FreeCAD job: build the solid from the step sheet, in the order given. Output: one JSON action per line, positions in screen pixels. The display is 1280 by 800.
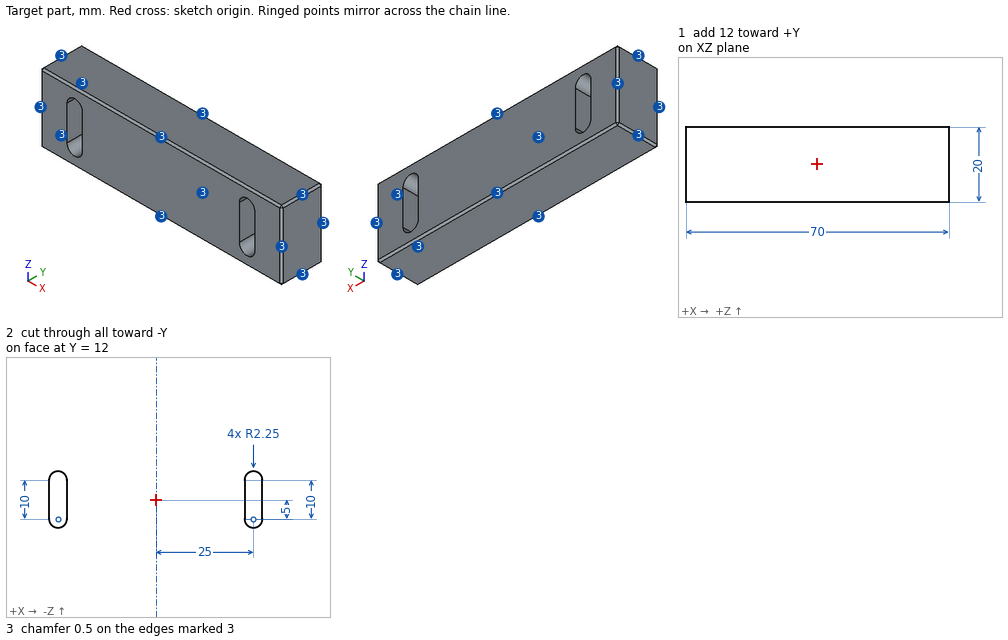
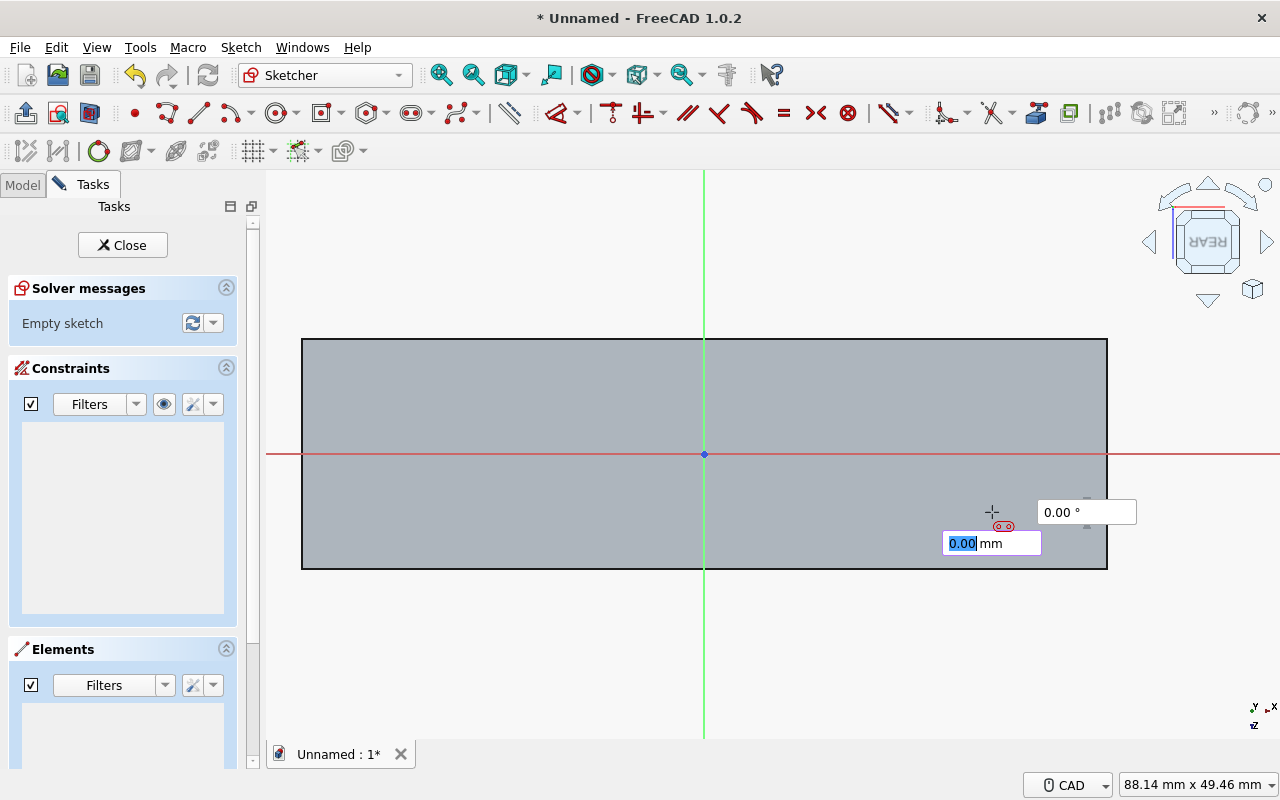
{"action": "left_click", "coordinate": [992, 396]}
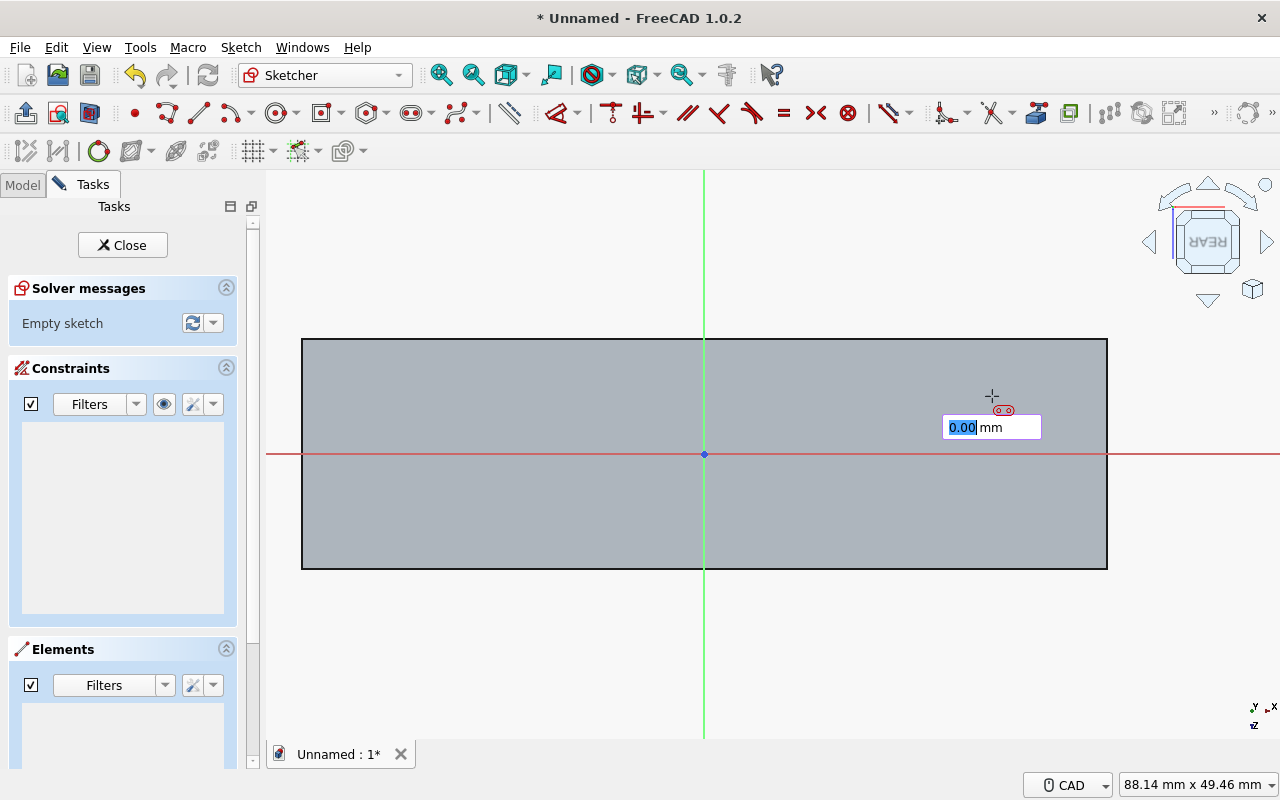
{"action": "left_click", "coordinate": [966, 437]}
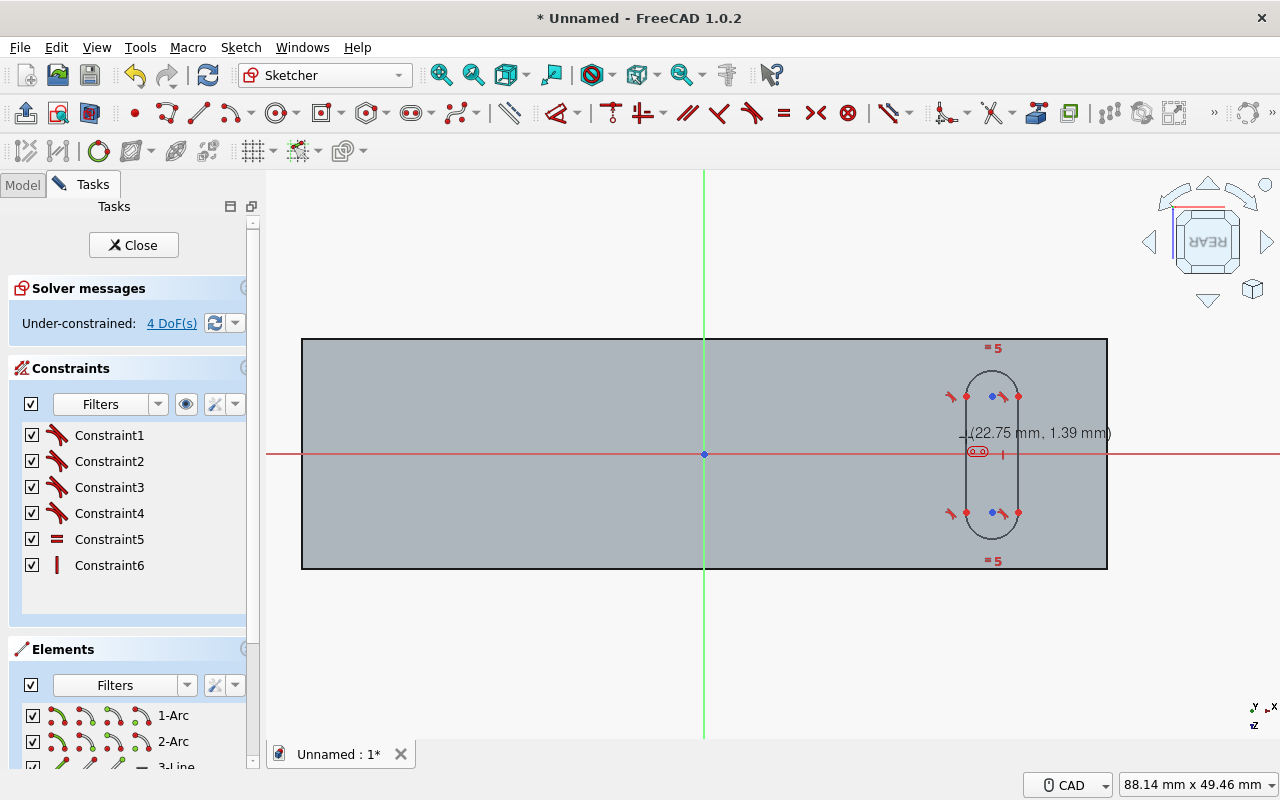
{"action": "left_click", "coordinate": [417, 512]}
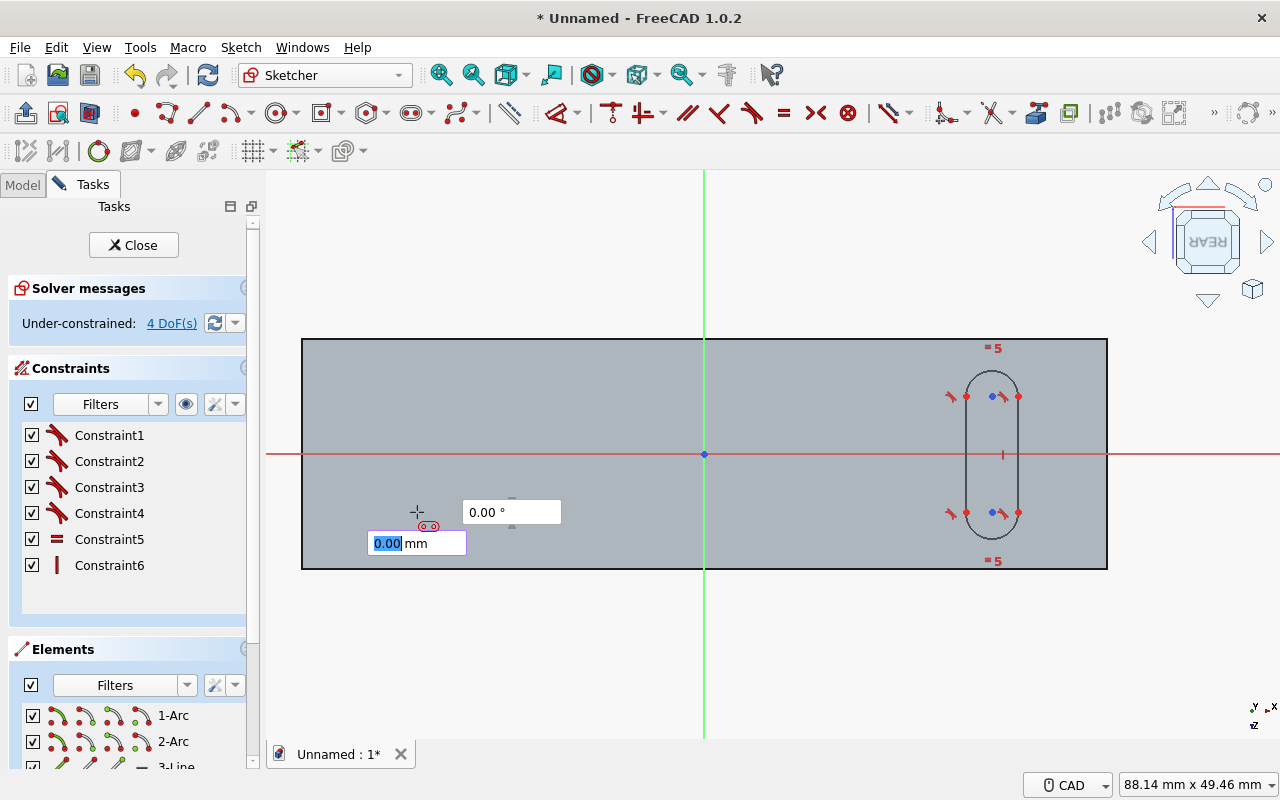
{"action": "left_click", "coordinate": [417, 396]}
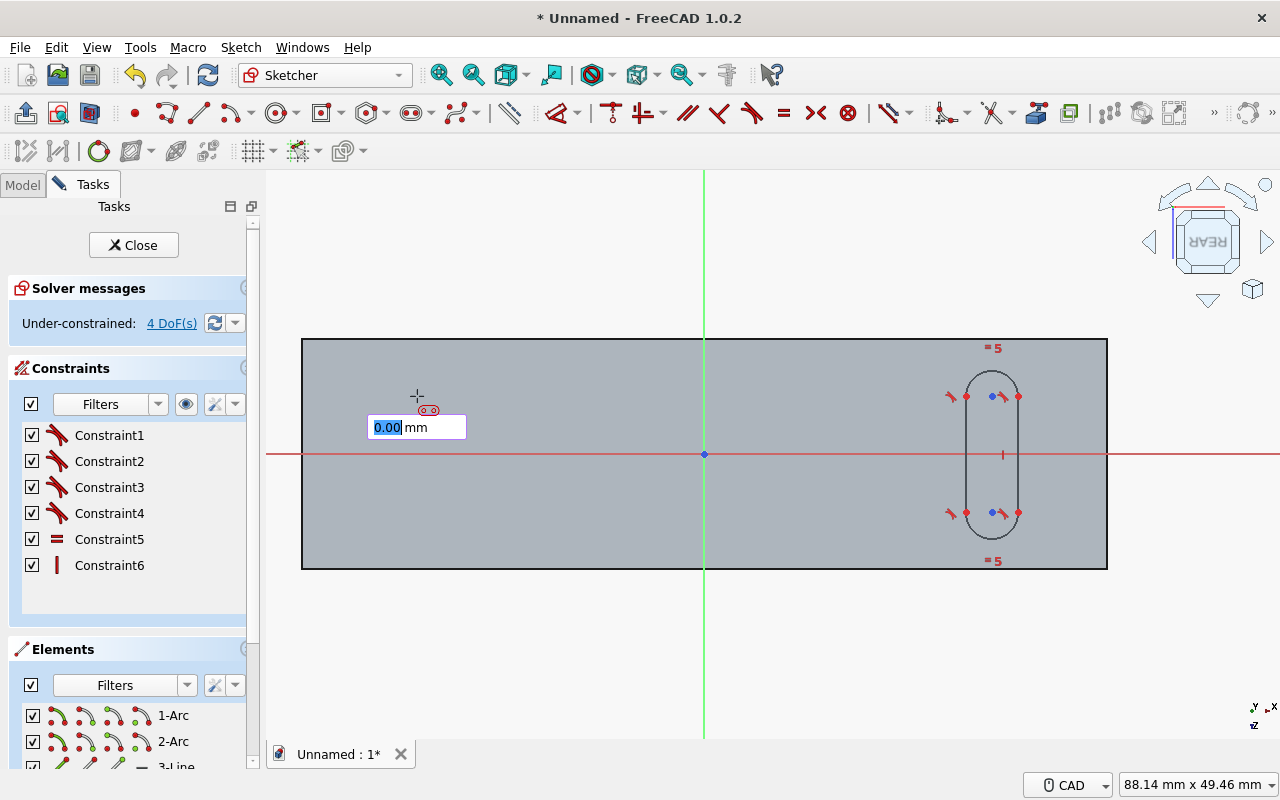
{"action": "left_click", "coordinate": [391, 437]}
{"action": "key", "text": "Escape"}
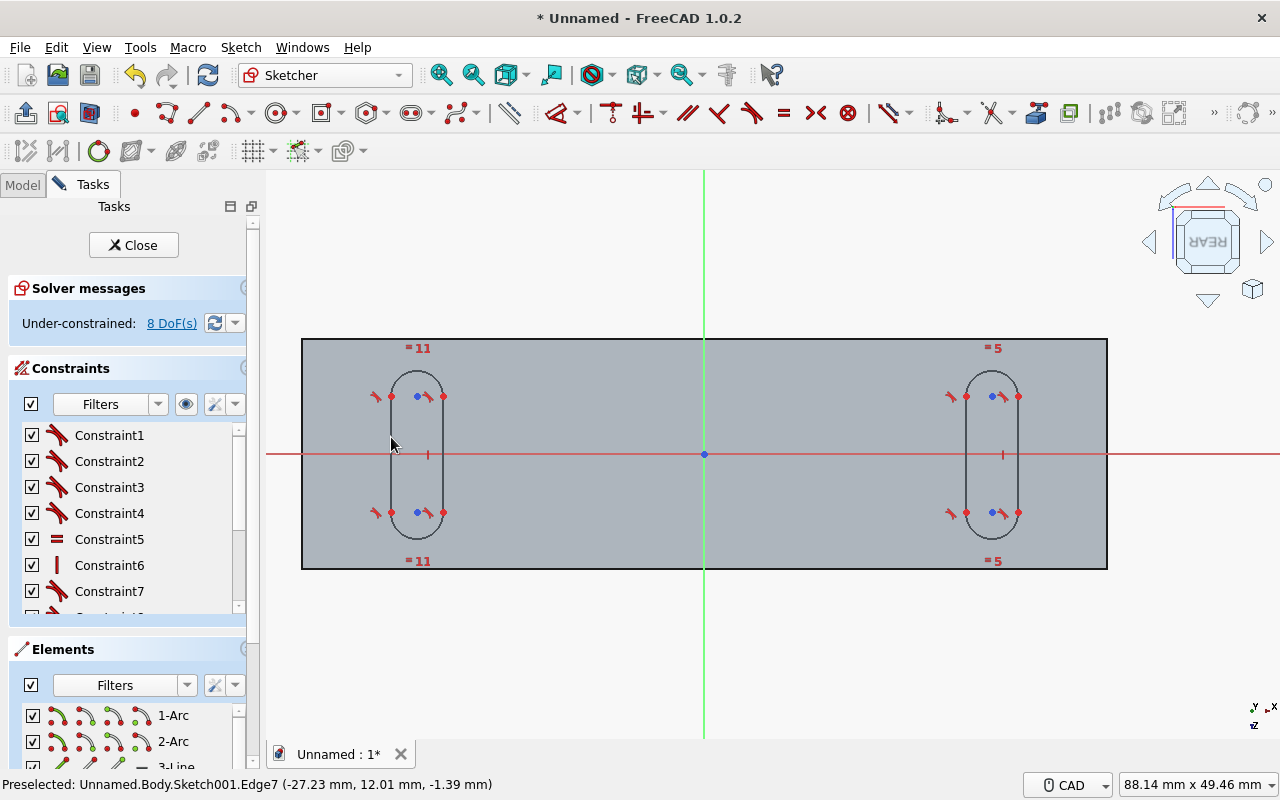
{"action": "left_click", "coordinate": [977, 534]}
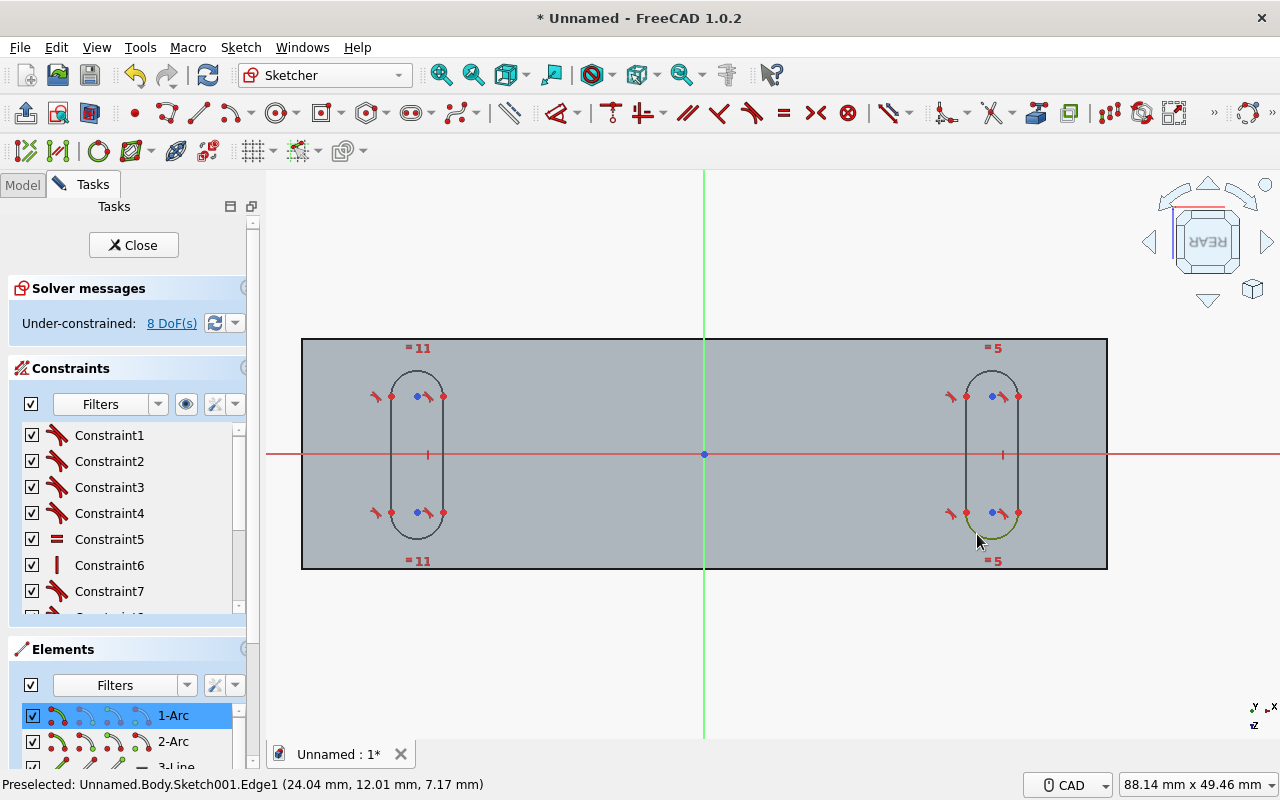
{"action": "left_click", "coordinate": [402, 534]}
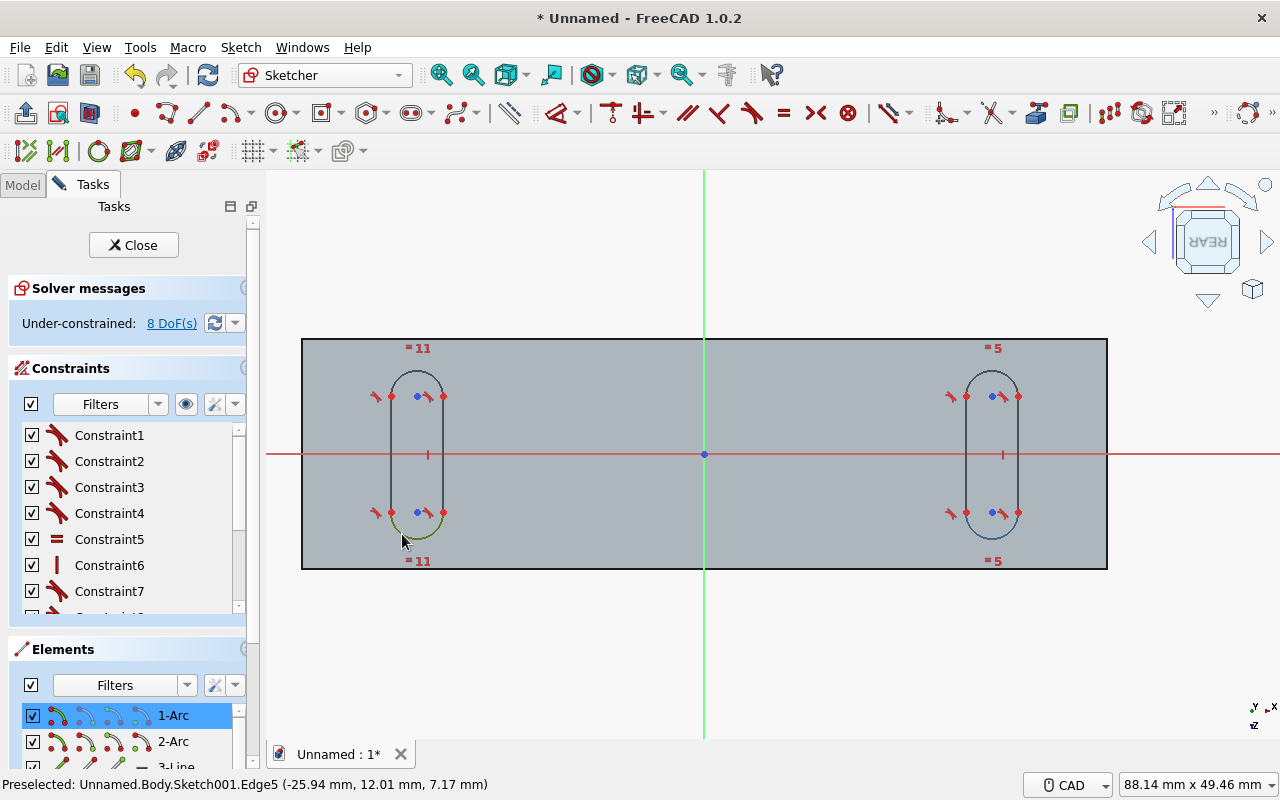
{"action": "left_click", "coordinate": [784, 114]}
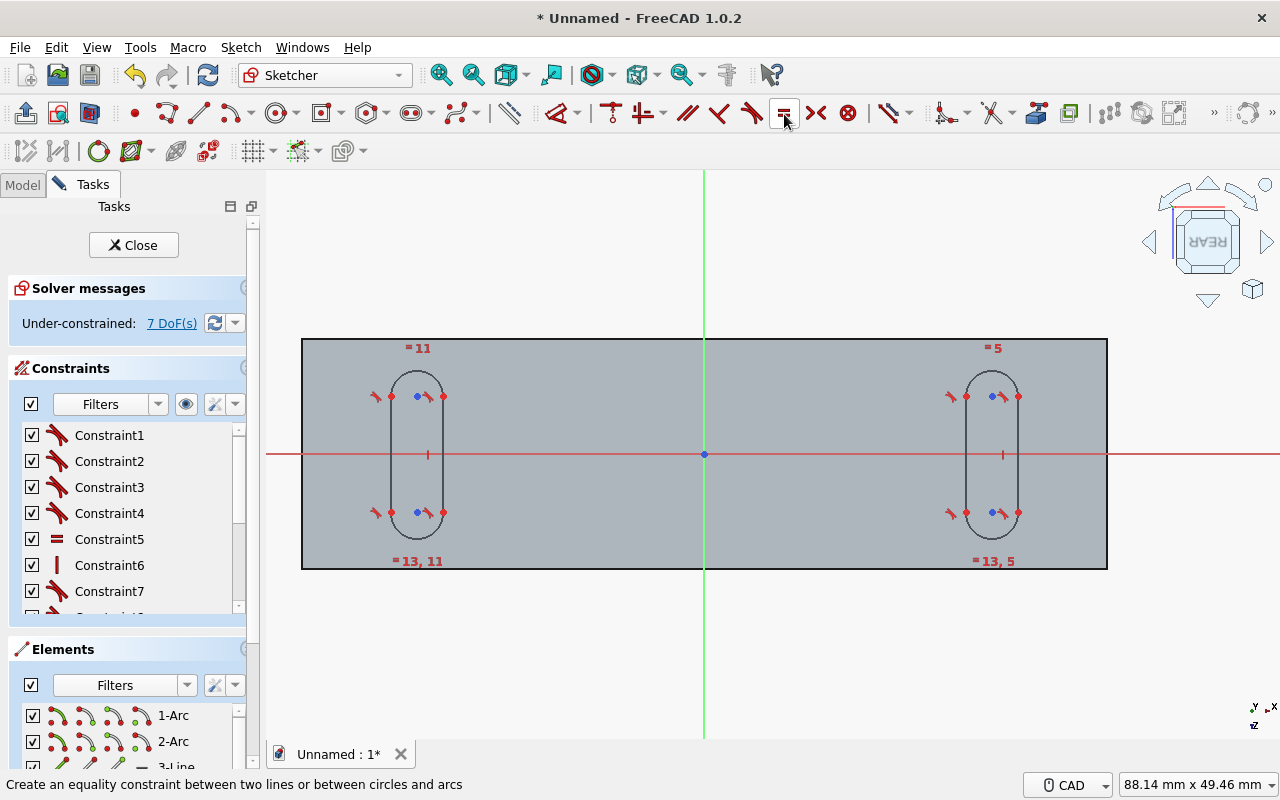
{"action": "left_click", "coordinate": [992, 513]}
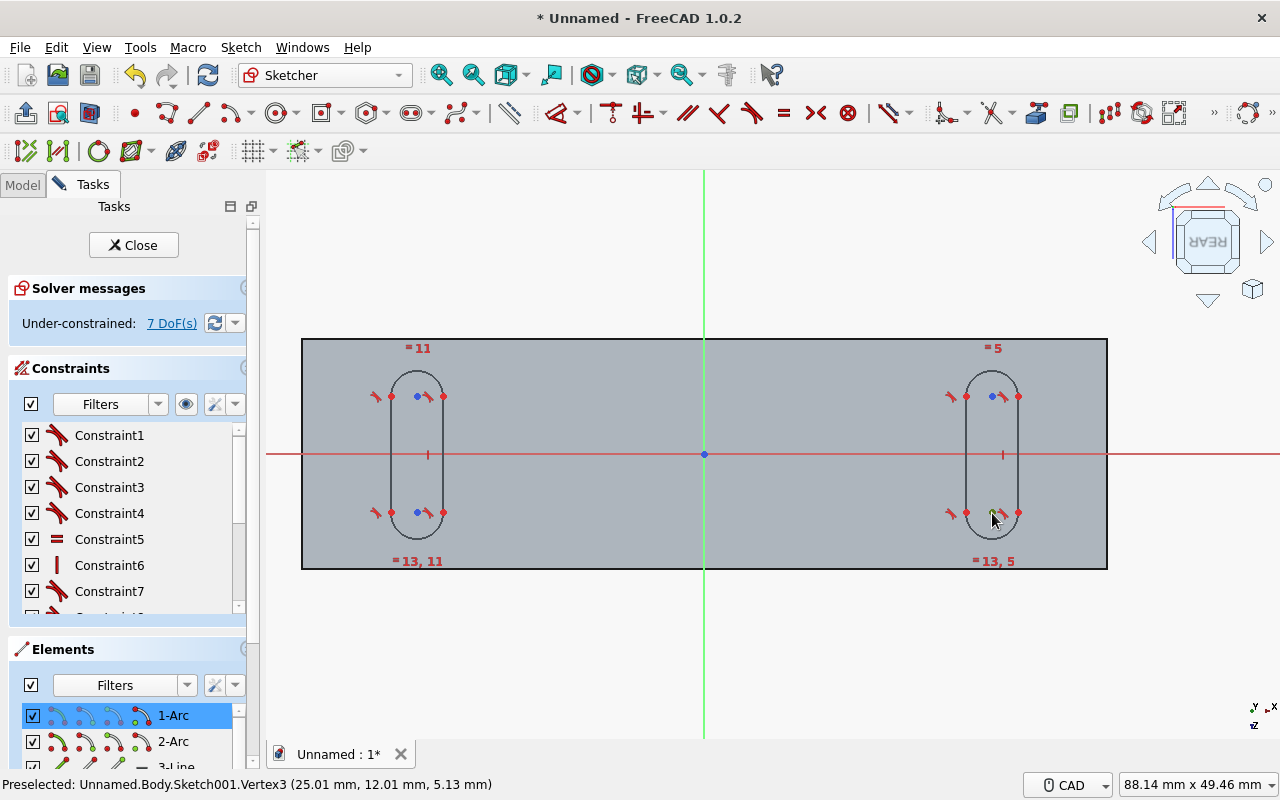
{"action": "left_click", "coordinate": [417, 513]}